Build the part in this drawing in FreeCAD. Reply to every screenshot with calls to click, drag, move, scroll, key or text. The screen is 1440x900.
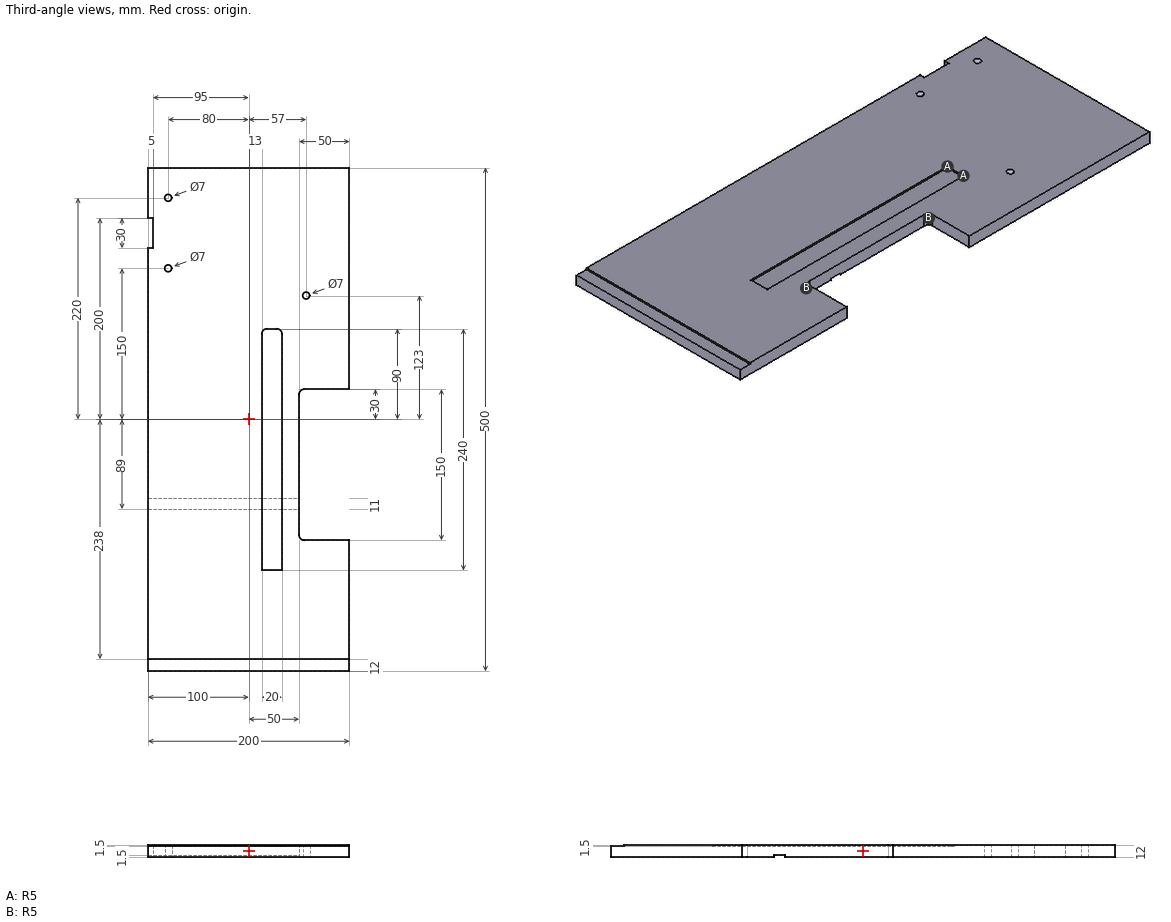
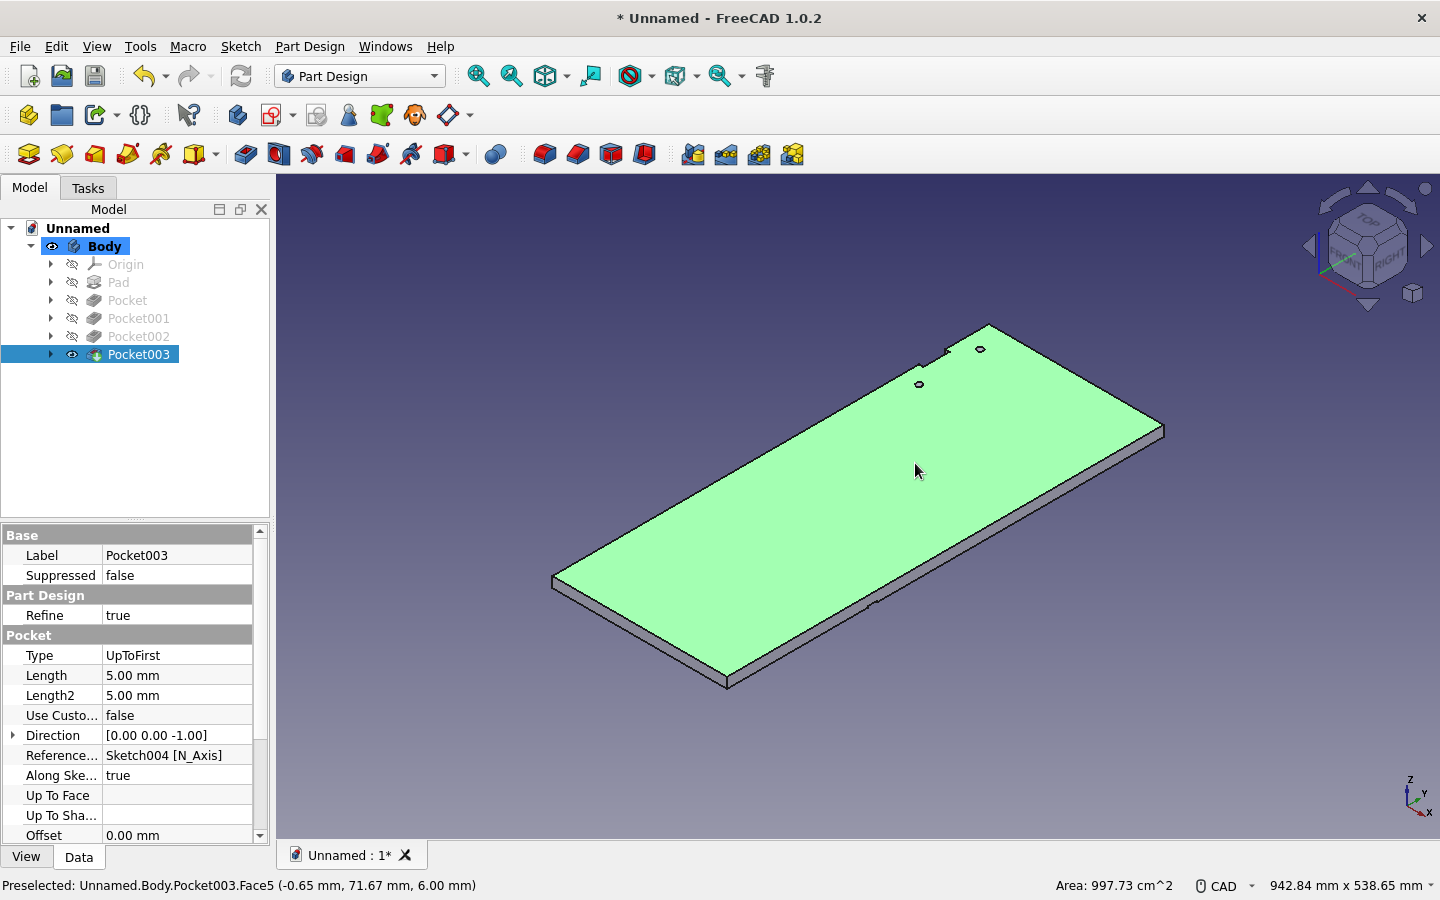
click(270, 116)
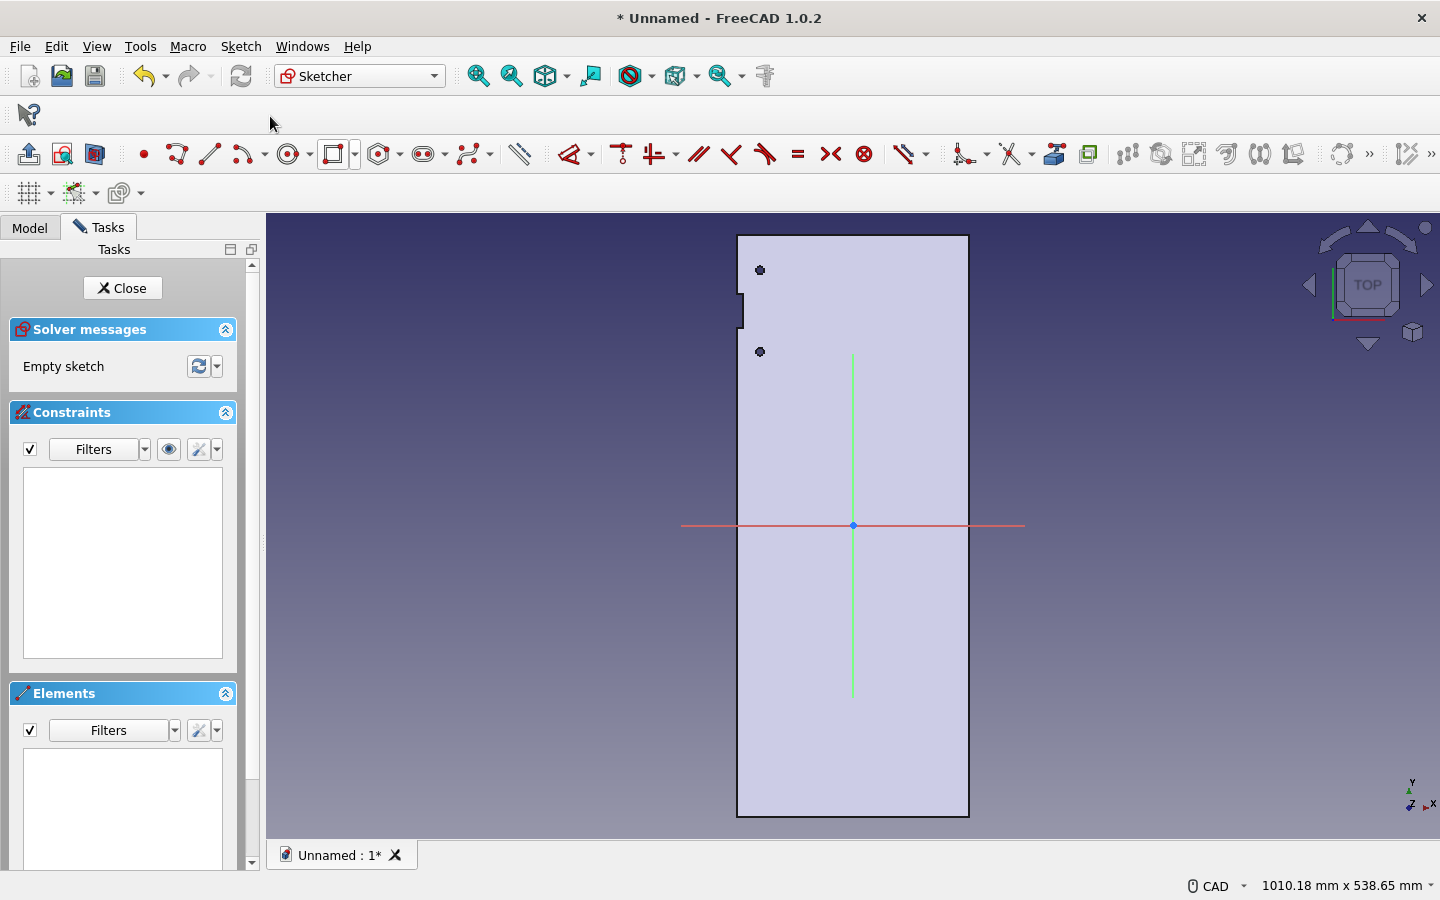
scroll(926, 376, up, 15)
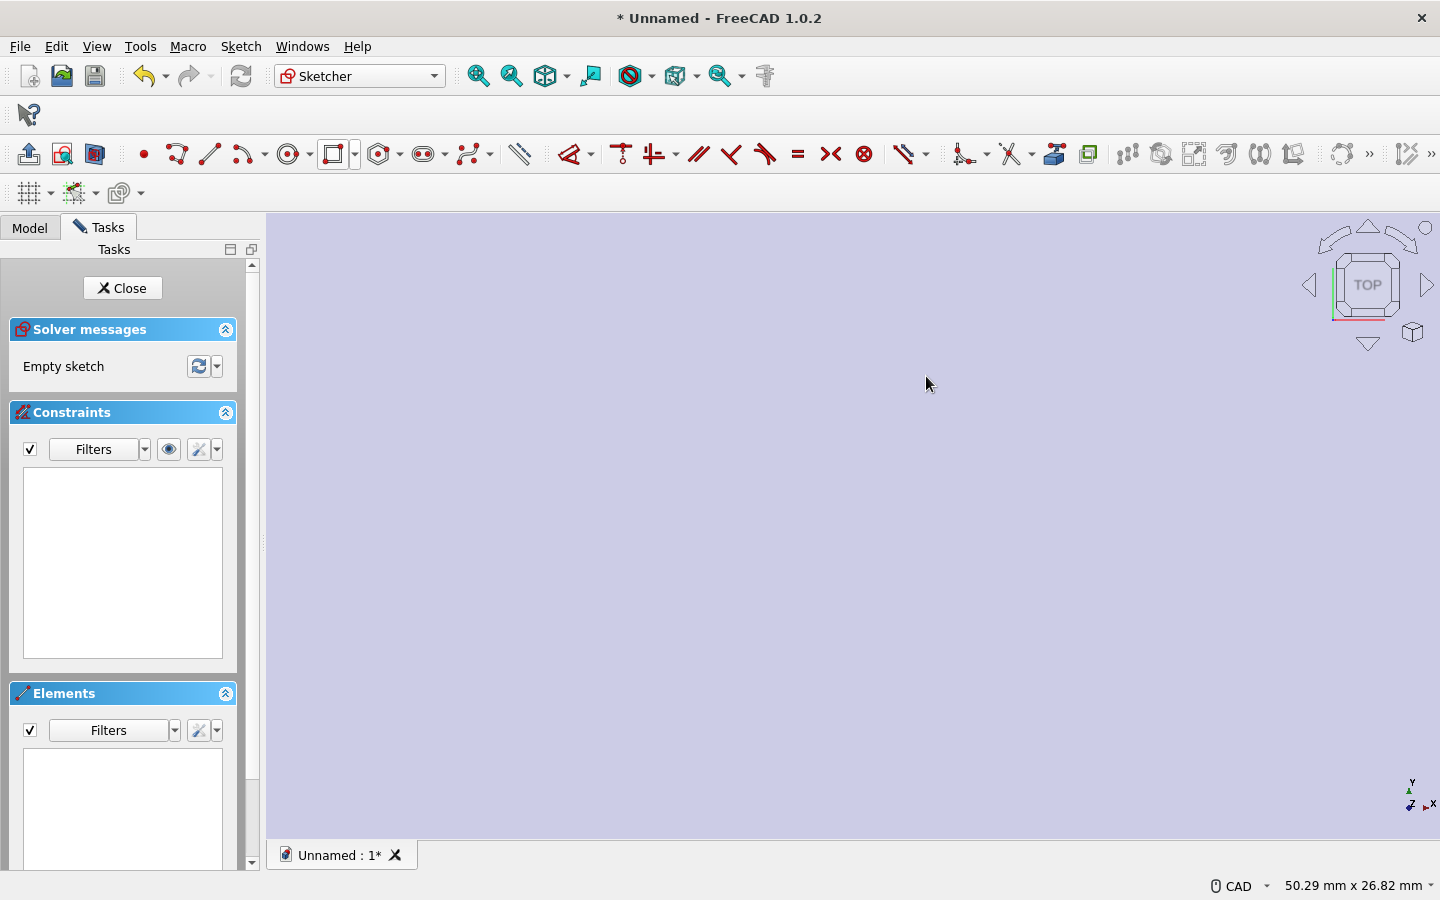
scroll(777, 505, up, 5)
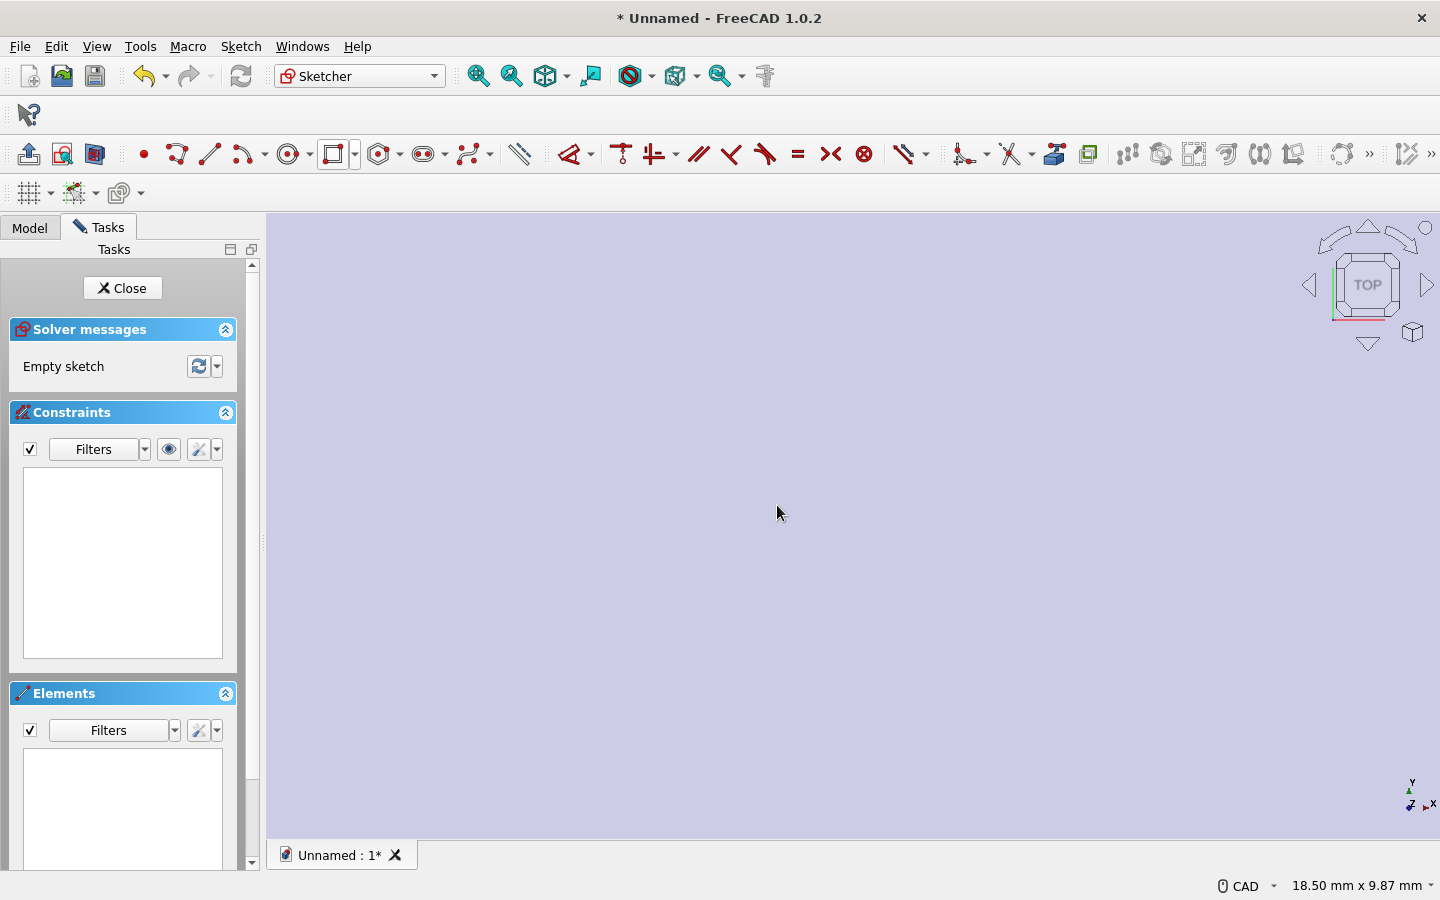
click(288, 154)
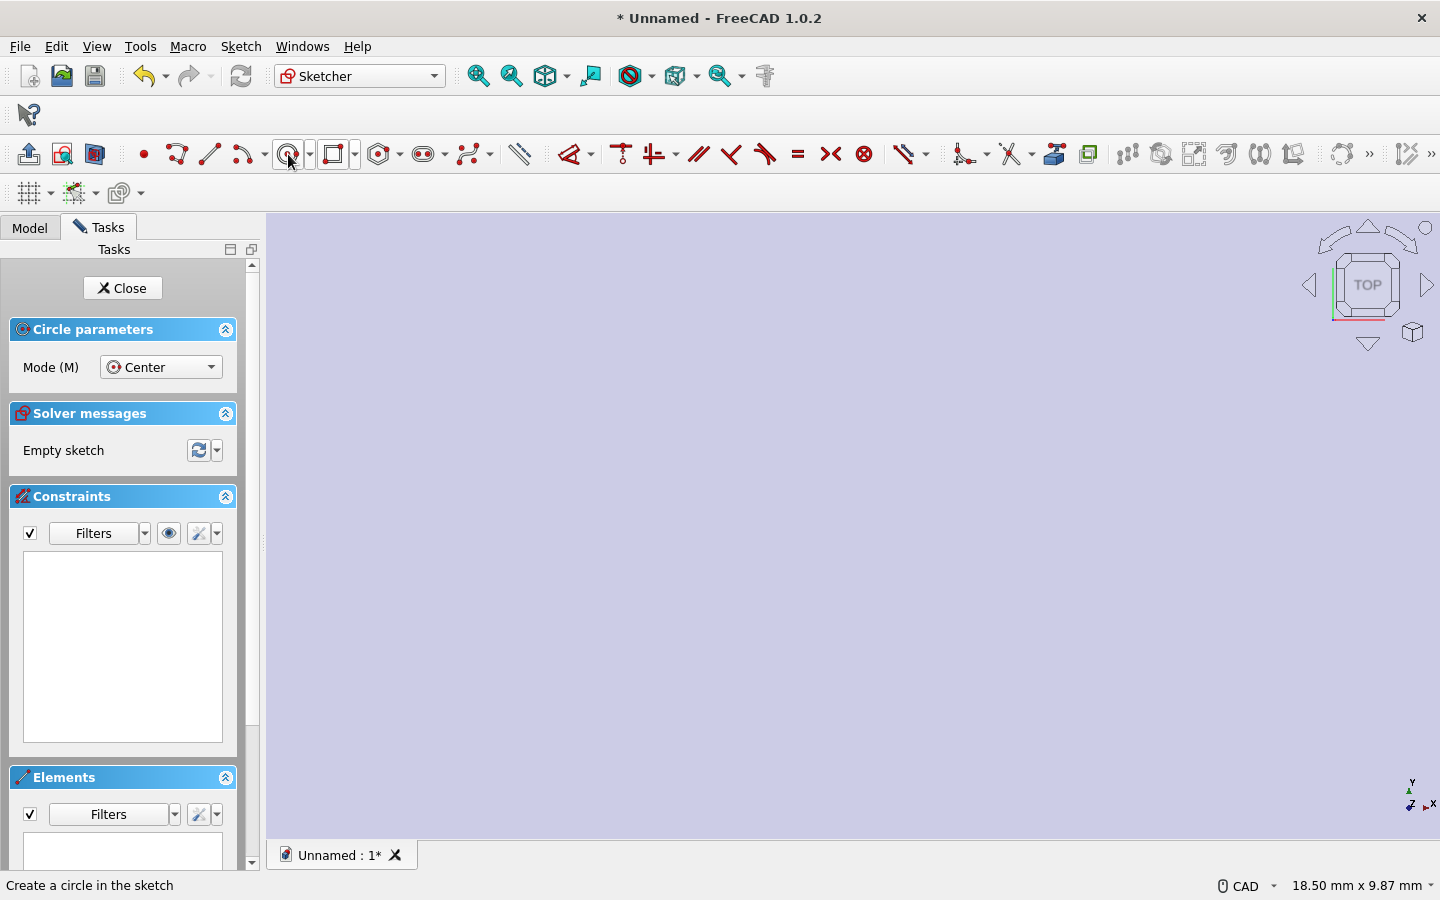
click(783, 525)
move(940, 368)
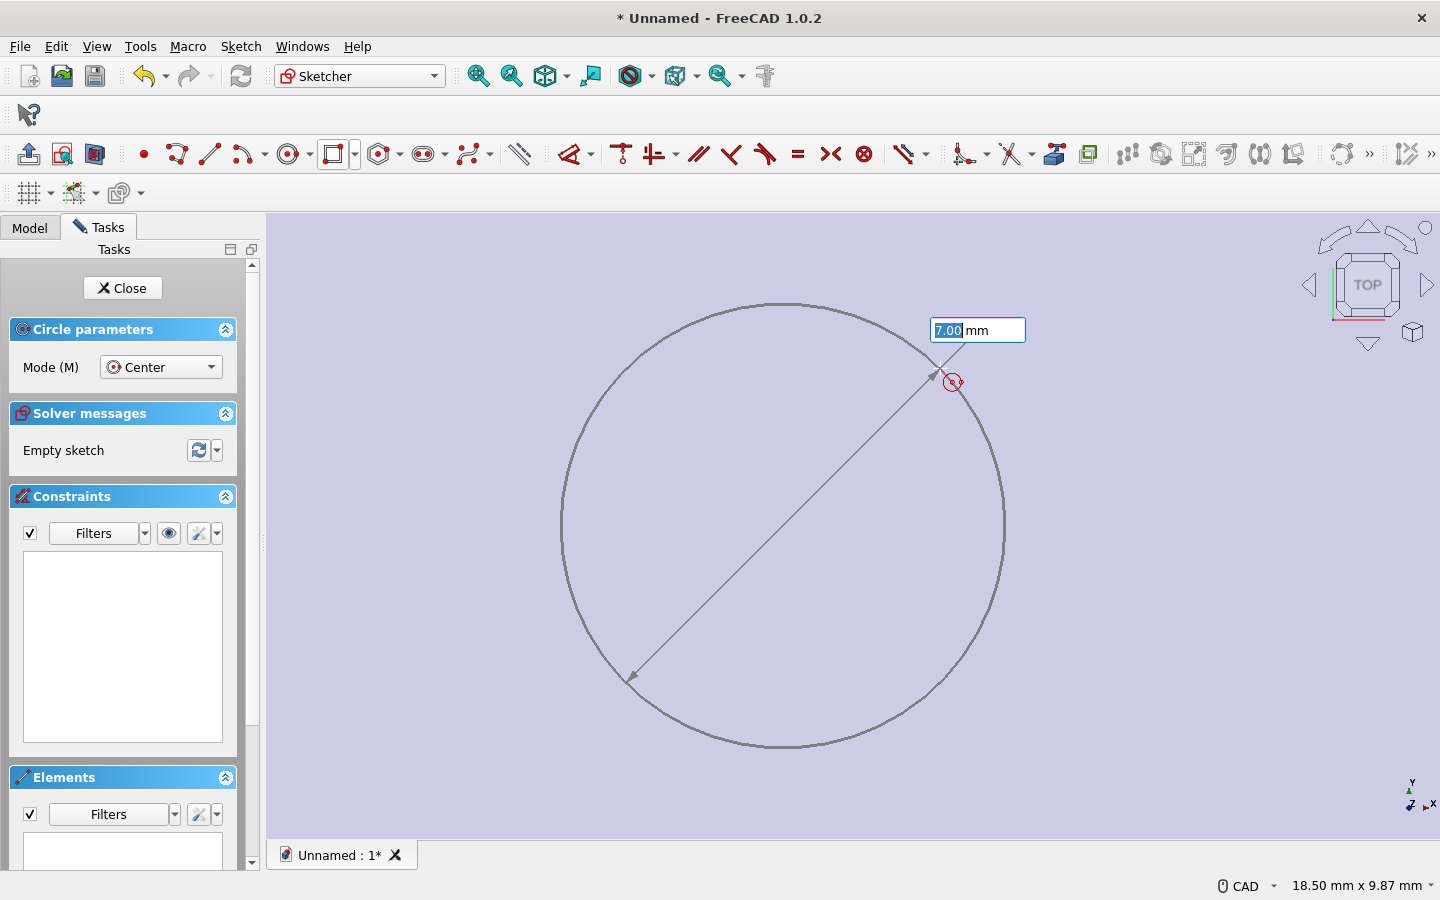
text(7)
key(Return)
key(Escape)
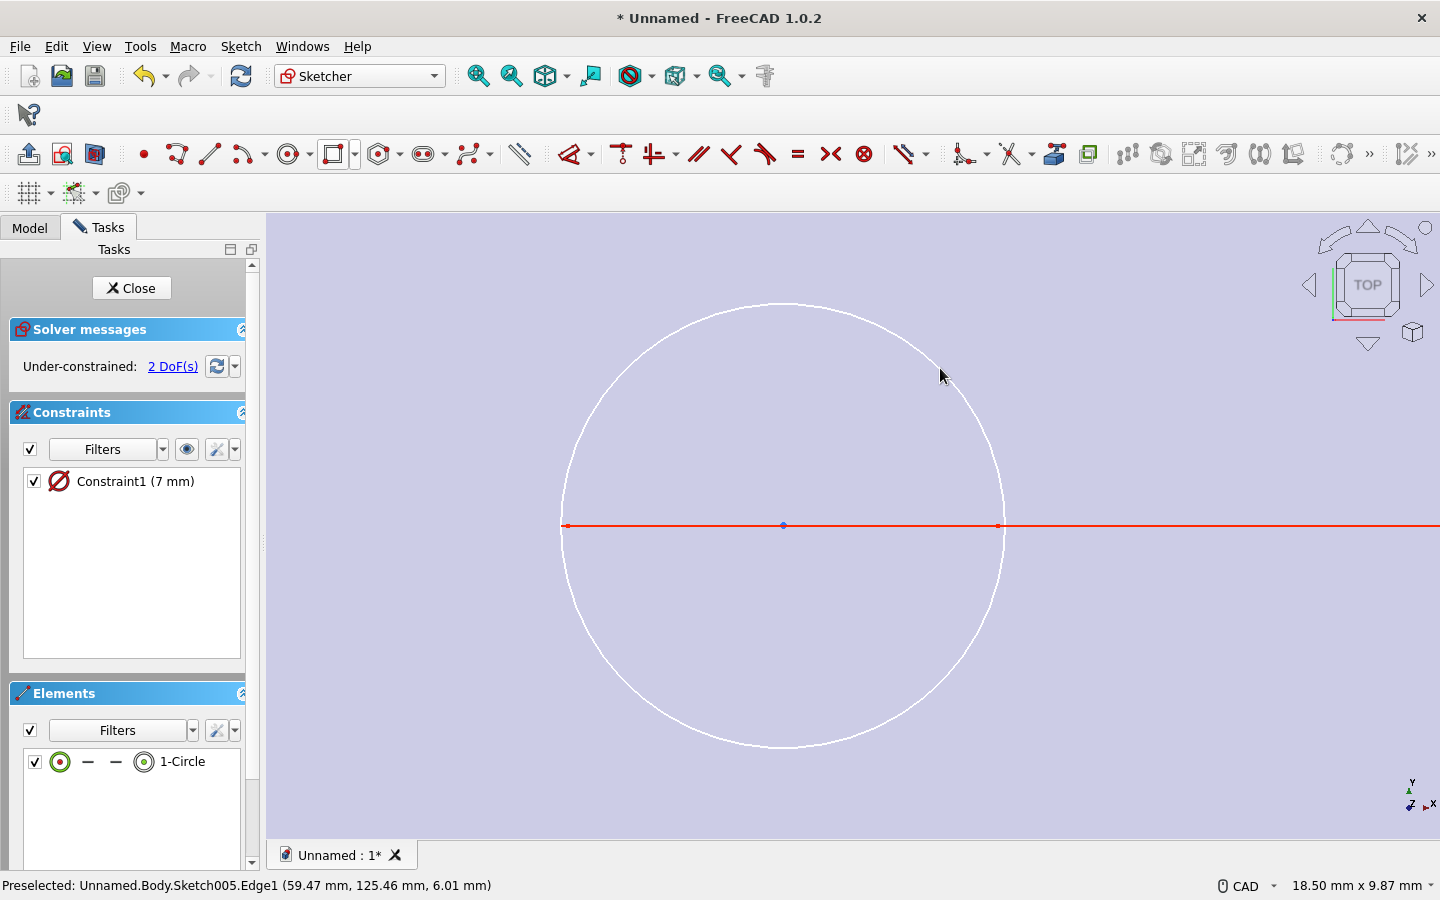
click(568, 154)